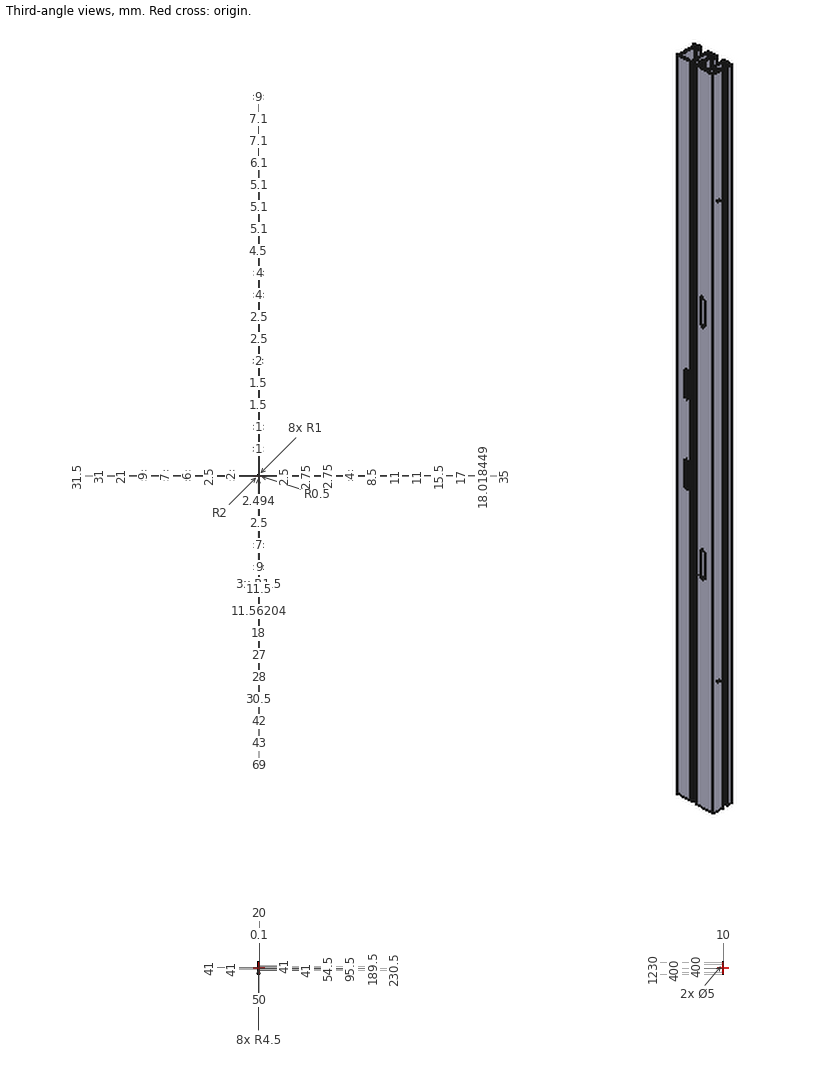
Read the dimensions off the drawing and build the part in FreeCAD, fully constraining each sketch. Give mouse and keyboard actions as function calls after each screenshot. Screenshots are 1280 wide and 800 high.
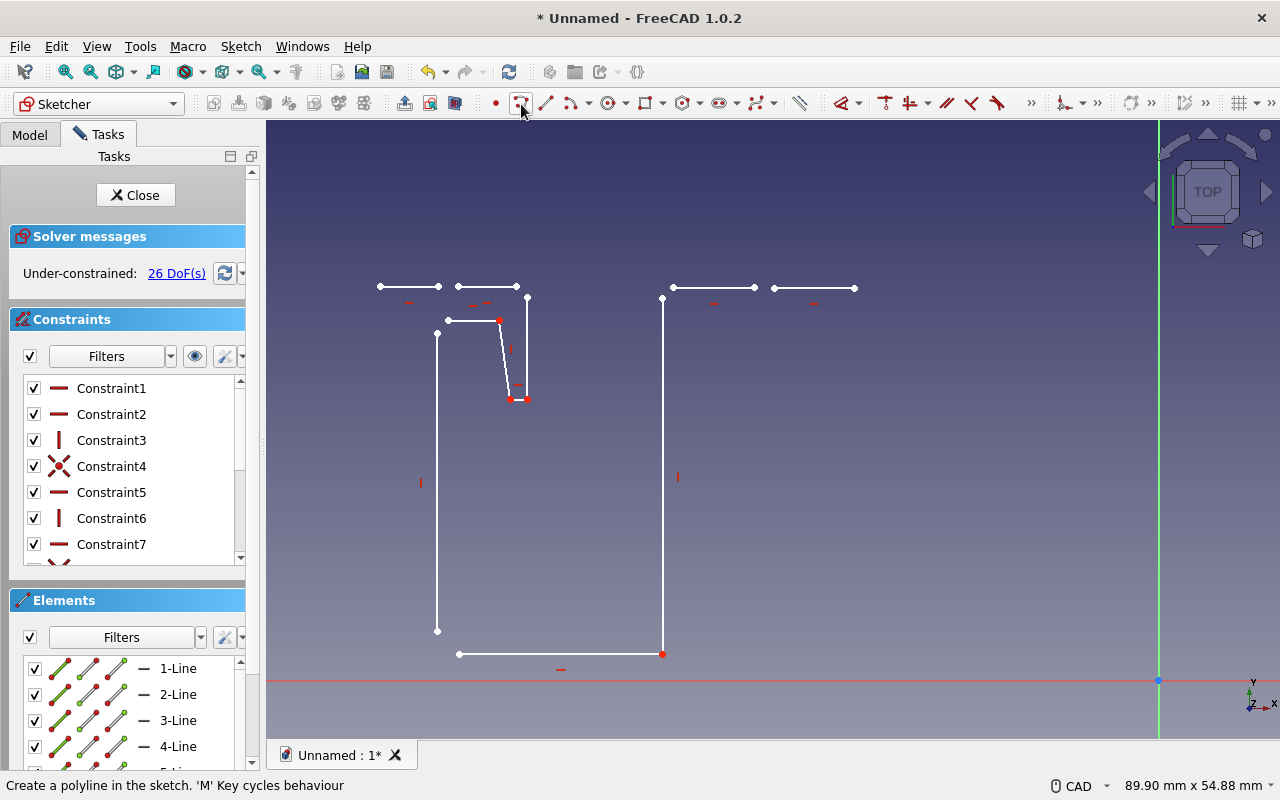
click(369, 297)
click(369, 320)
click(392, 320)
right_click(392, 320)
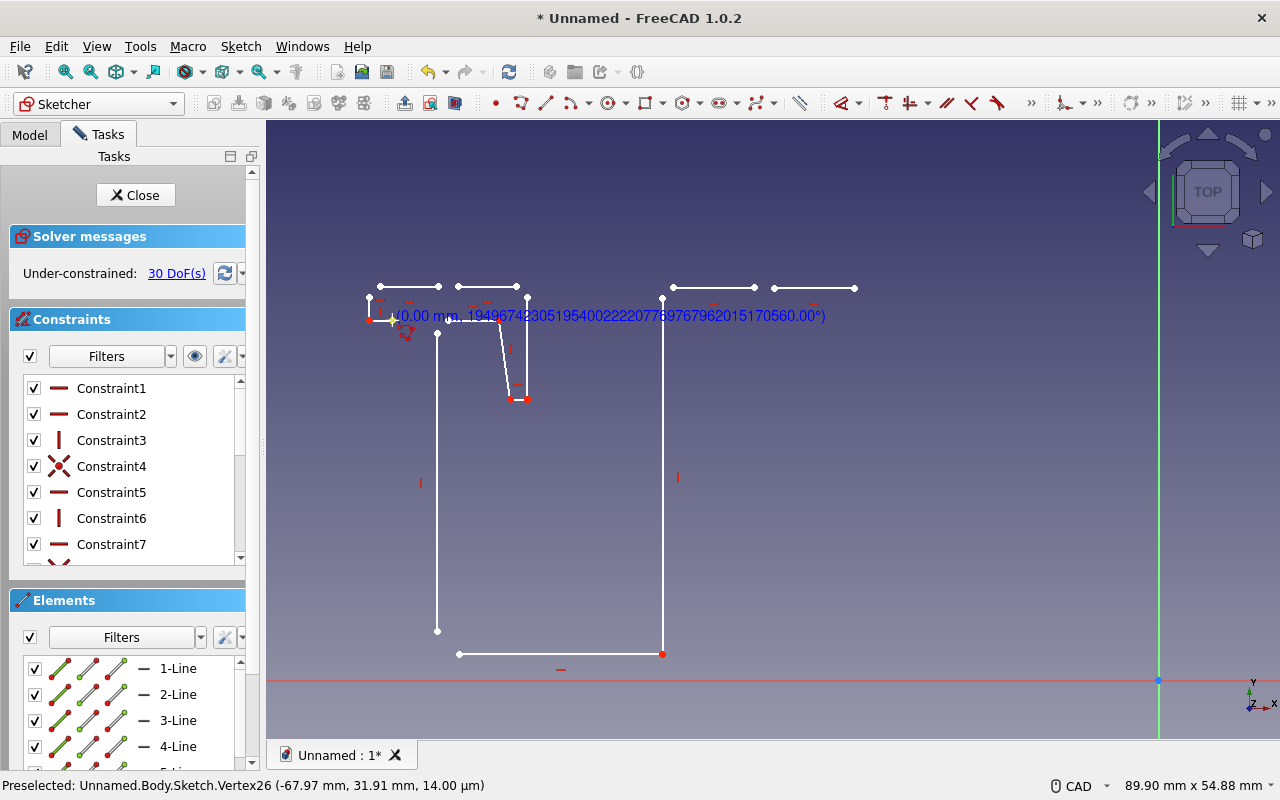
click(403, 331)
click(403, 681)
click(719, 672)
click(719, 653)
click(691, 653)
click(691, 585)
click(843, 585)
click(843, 653)
click(815, 653)
click(815, 681)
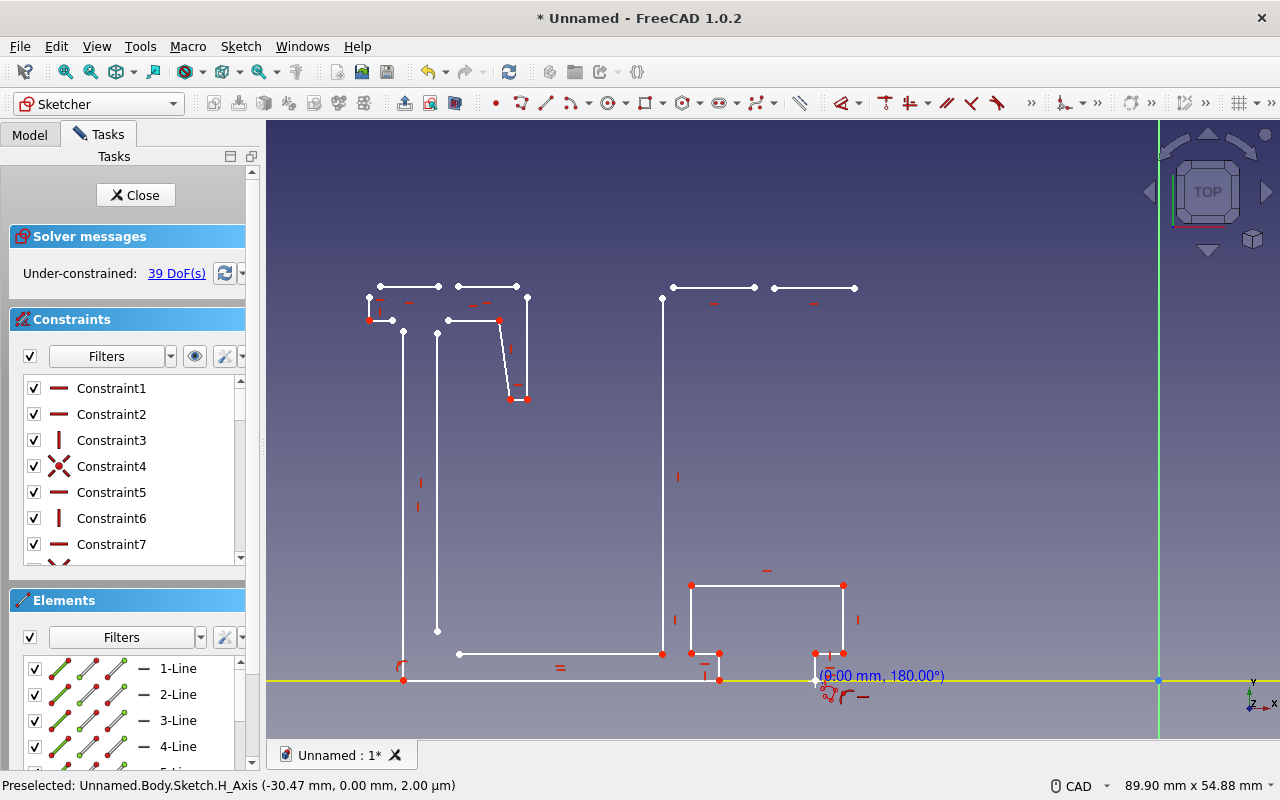
scroll(584, 320, down, 2)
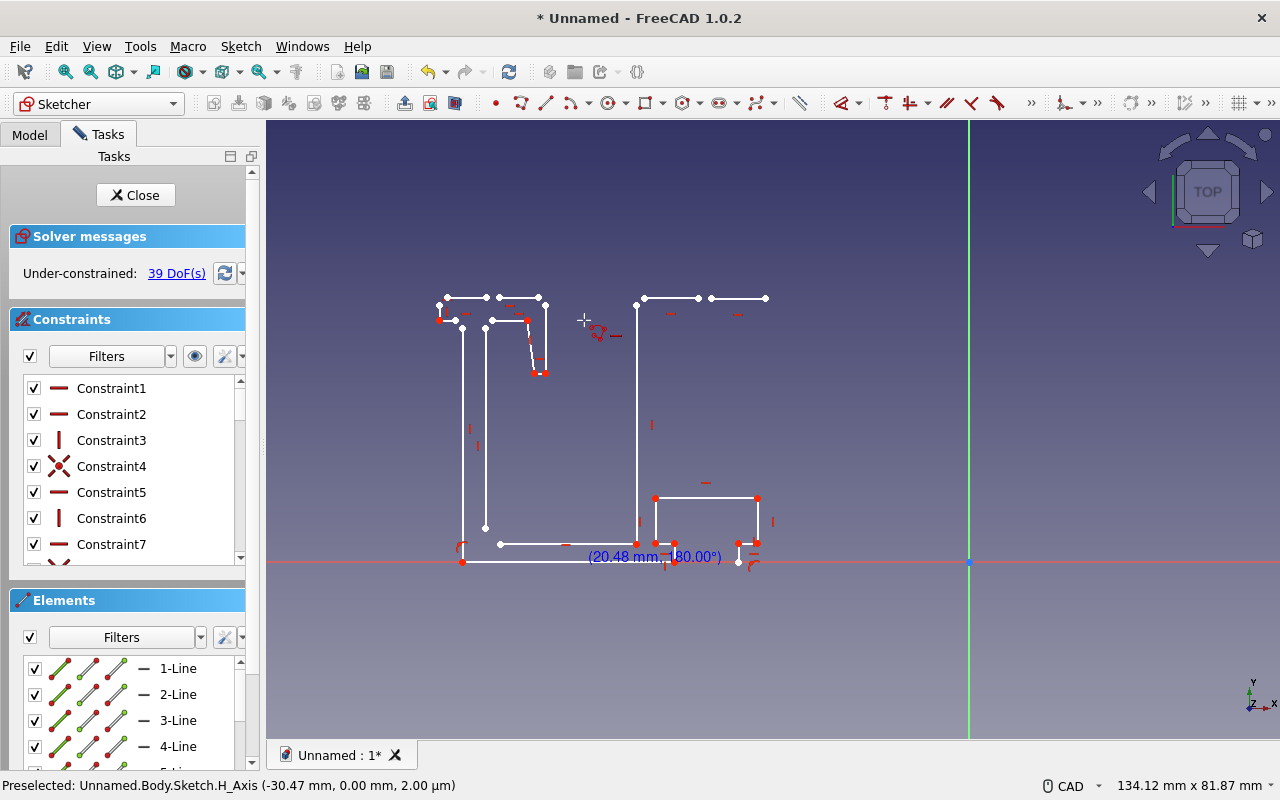
click(969, 562)
click(960, 424)
click(950, 424)
click(950, 445)
click(882, 445)
click(882, 328)
right_click(882, 328)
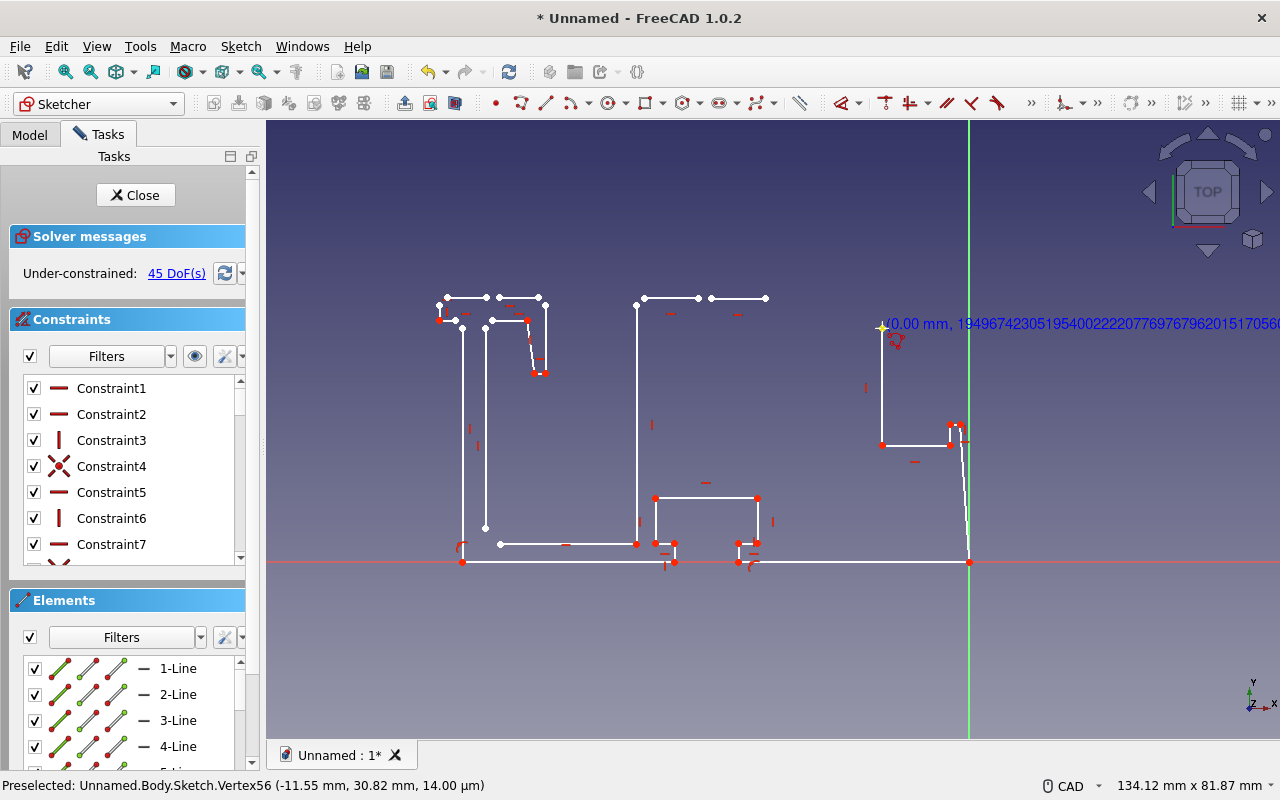
scroll(890, 320, up, 2)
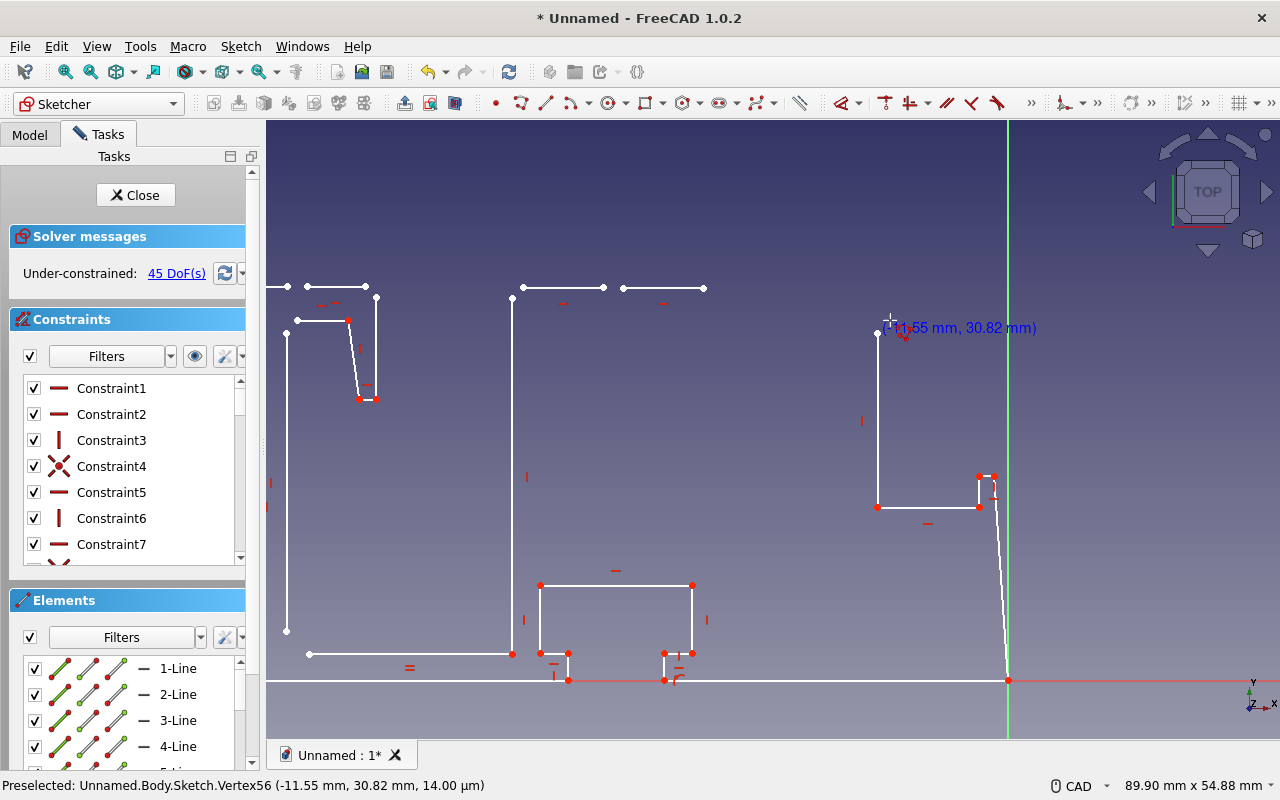
click(890, 320)
click(935, 320)
click(935, 348)
click(980, 348)
click(980, 379)
click(1008, 379)
click(999, 286)
click(939, 286)
right_click(939, 286)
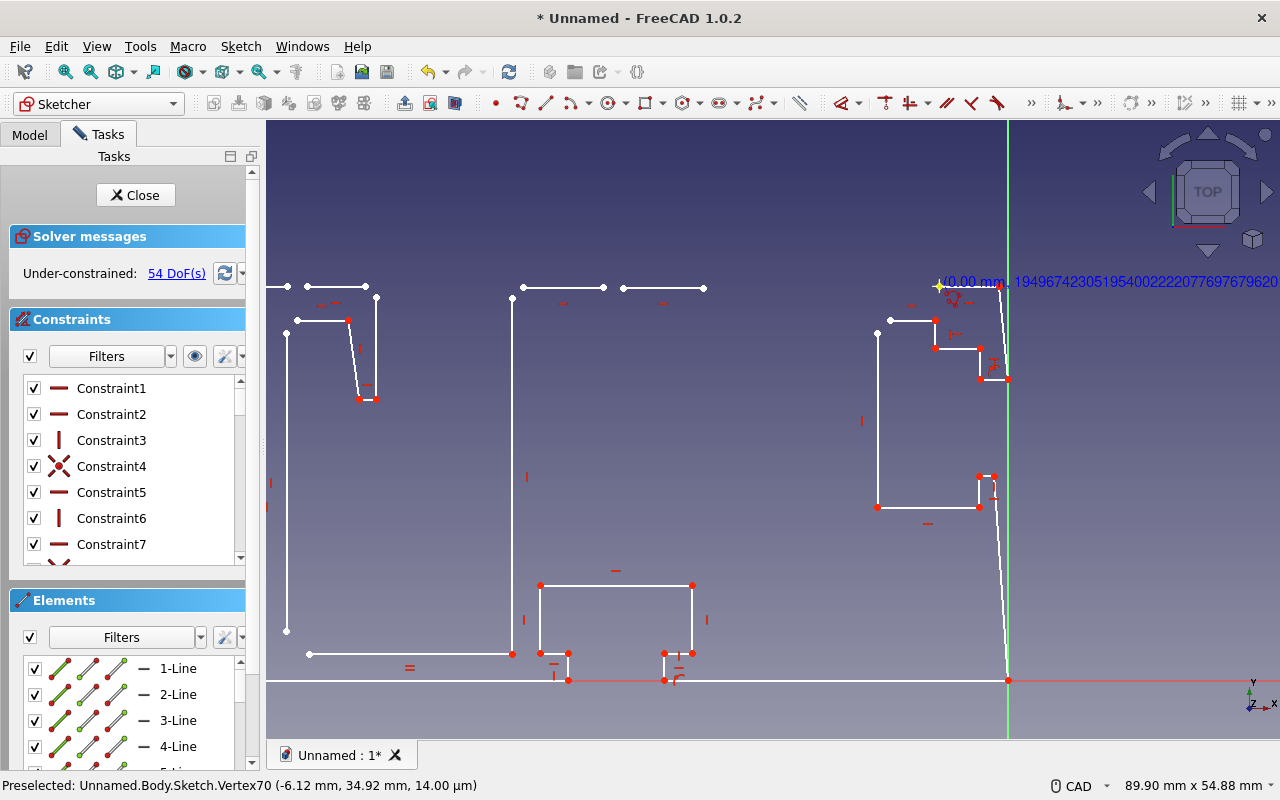
click(546, 104)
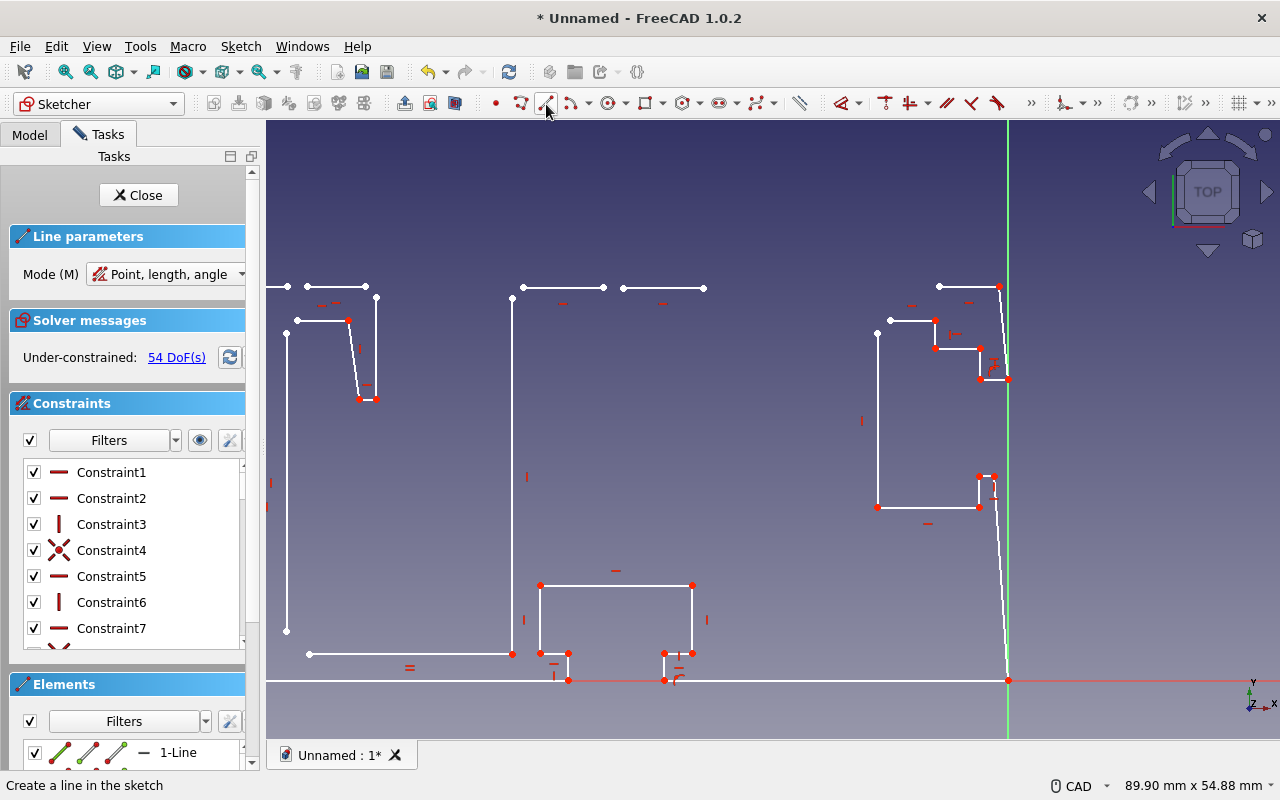
click(919, 286)
click(861, 286)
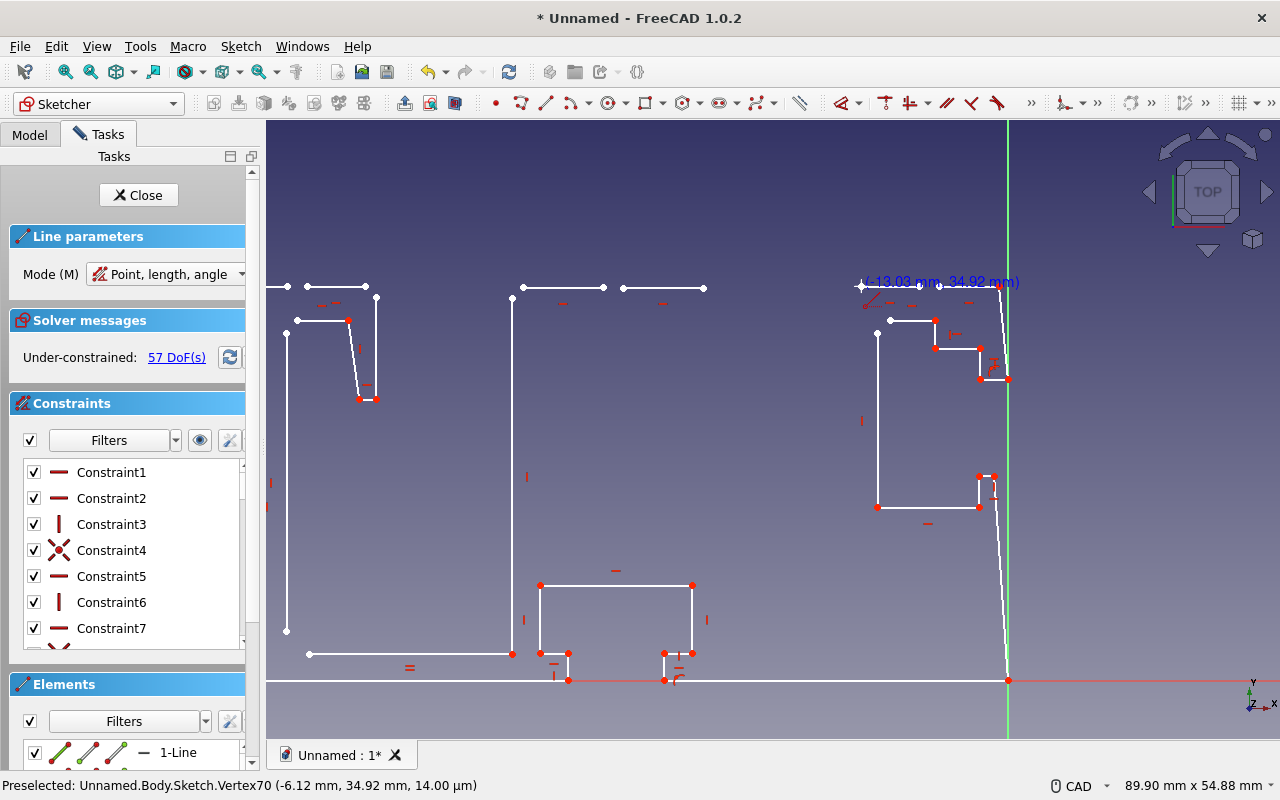
click(521, 104)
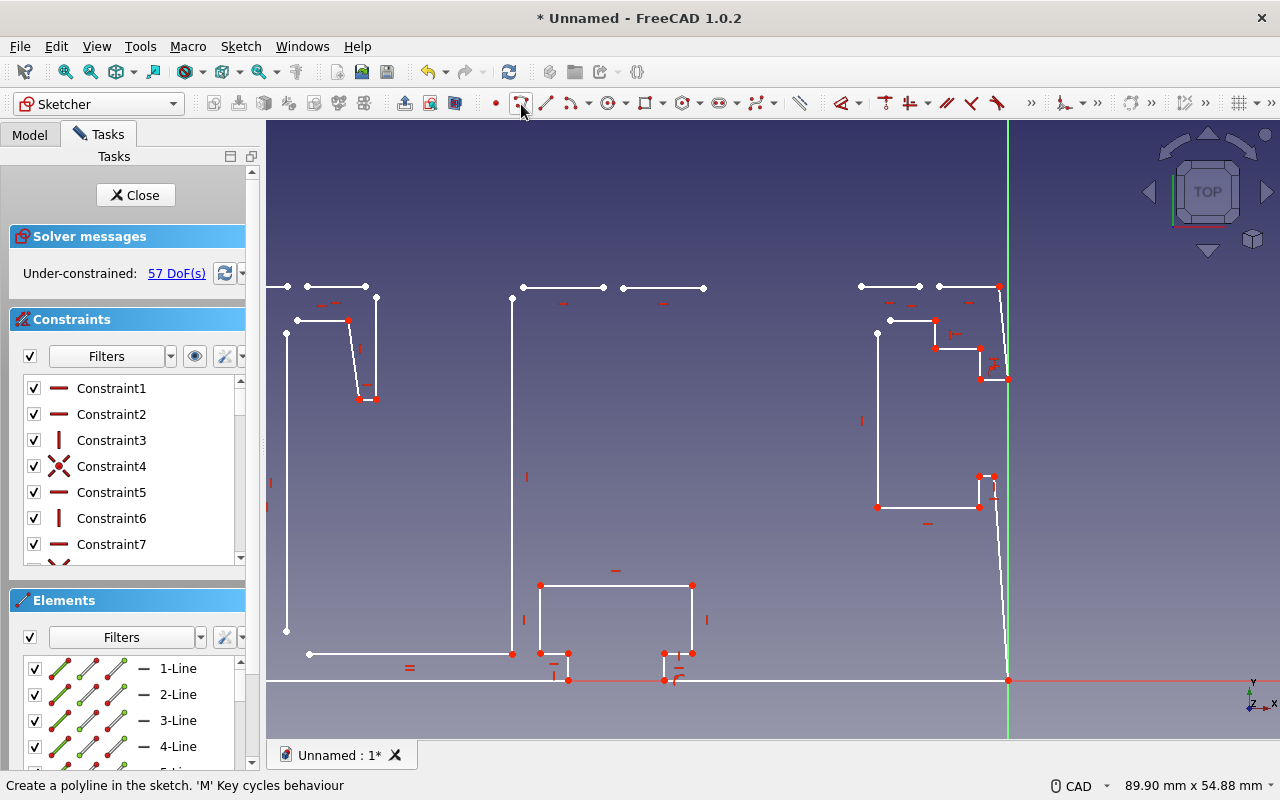
click(850, 297)
click(850, 653)
click(720, 653)
click(720, 557)
click(658, 512)
click(658, 320)
click(687, 320)
click(698, 399)
click(715, 399)
click(715, 297)
right_click(715, 297)